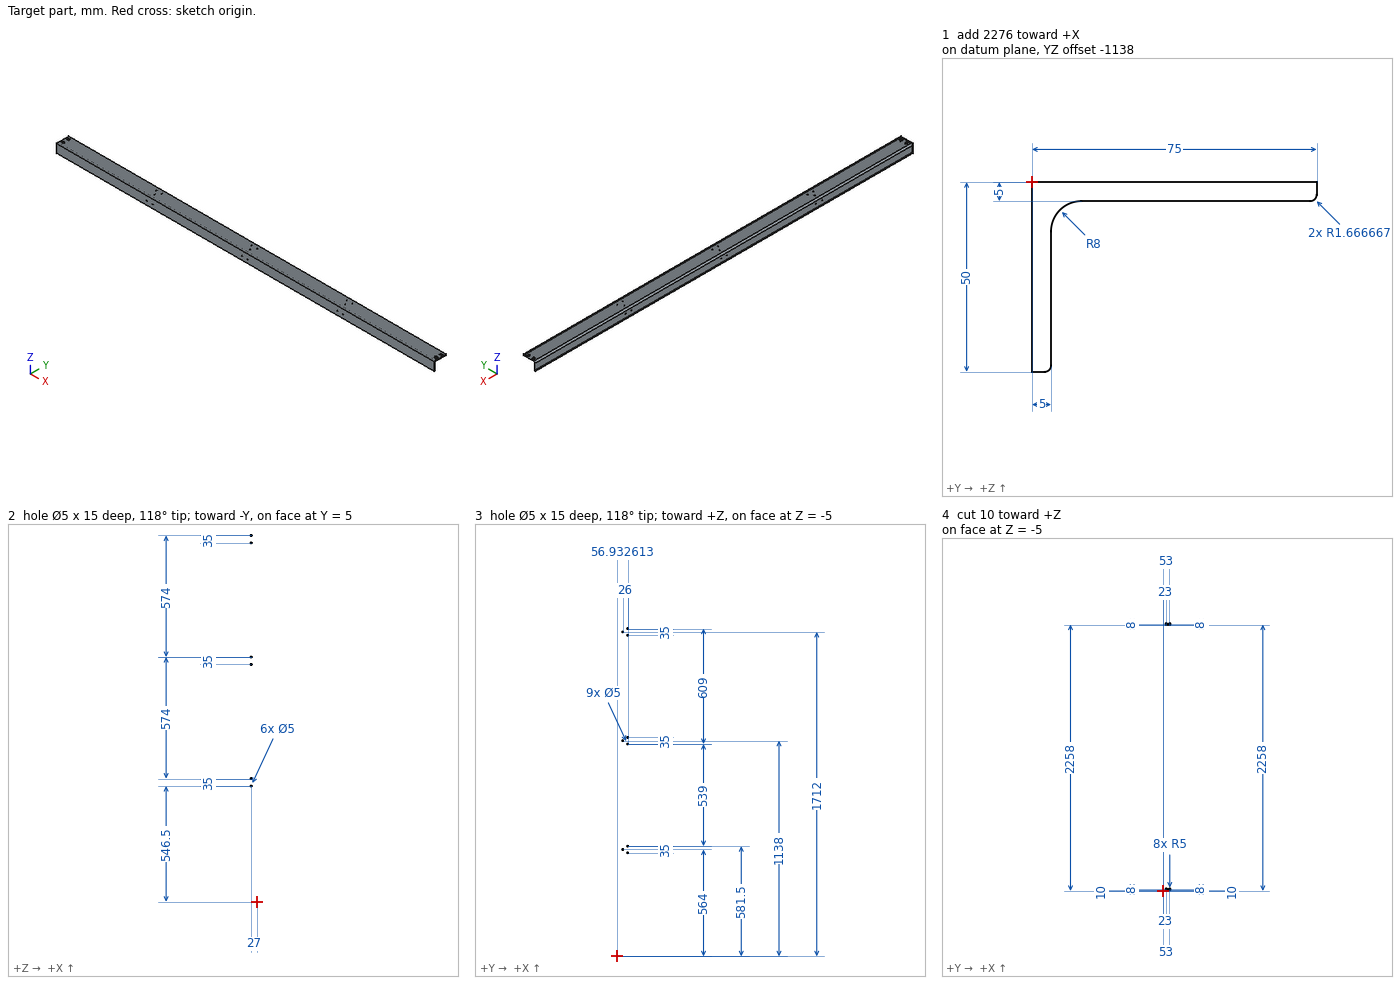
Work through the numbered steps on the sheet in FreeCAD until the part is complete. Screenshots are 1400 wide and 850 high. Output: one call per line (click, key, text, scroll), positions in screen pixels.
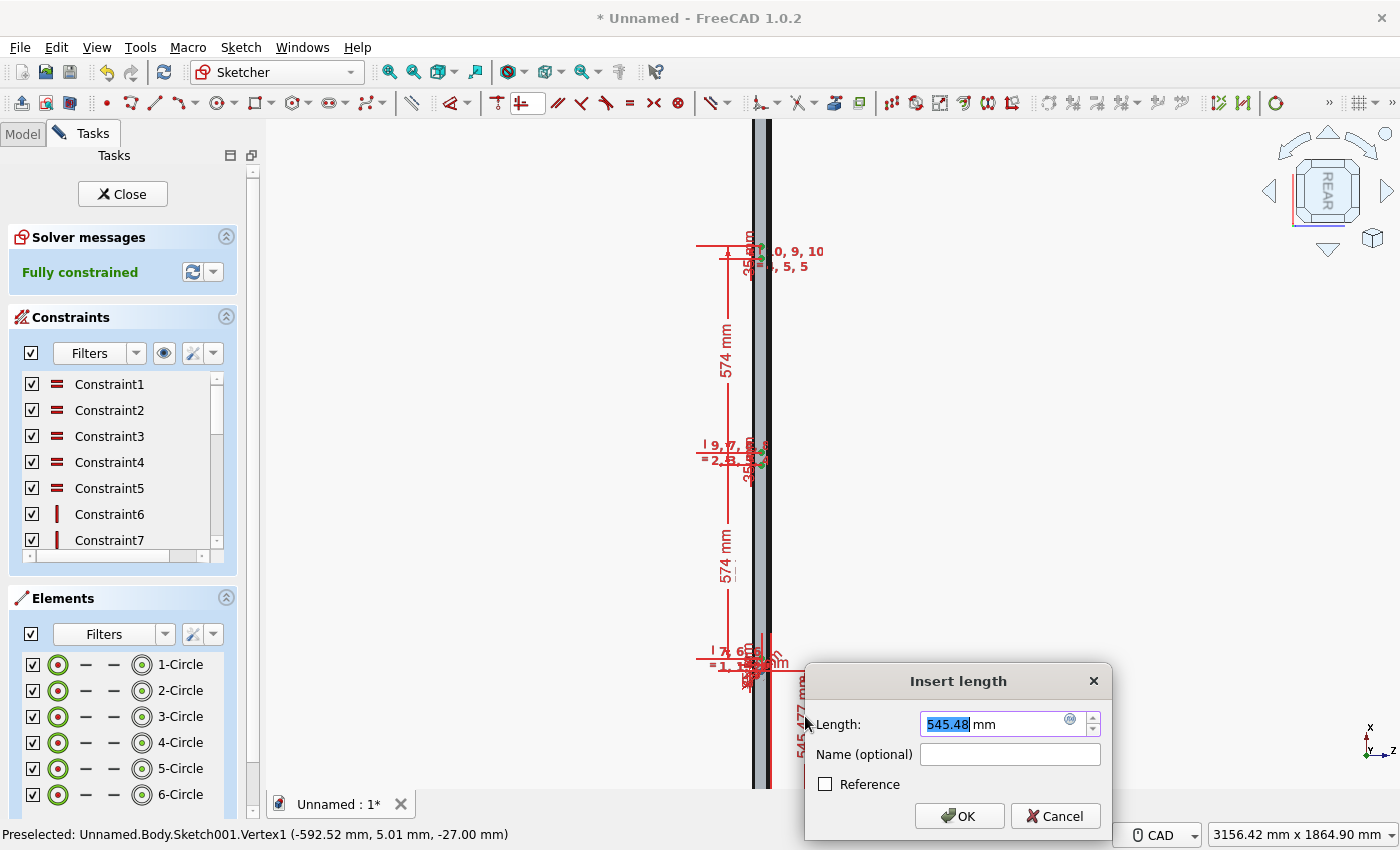
text(546.5)
key(Return)
key(Escape)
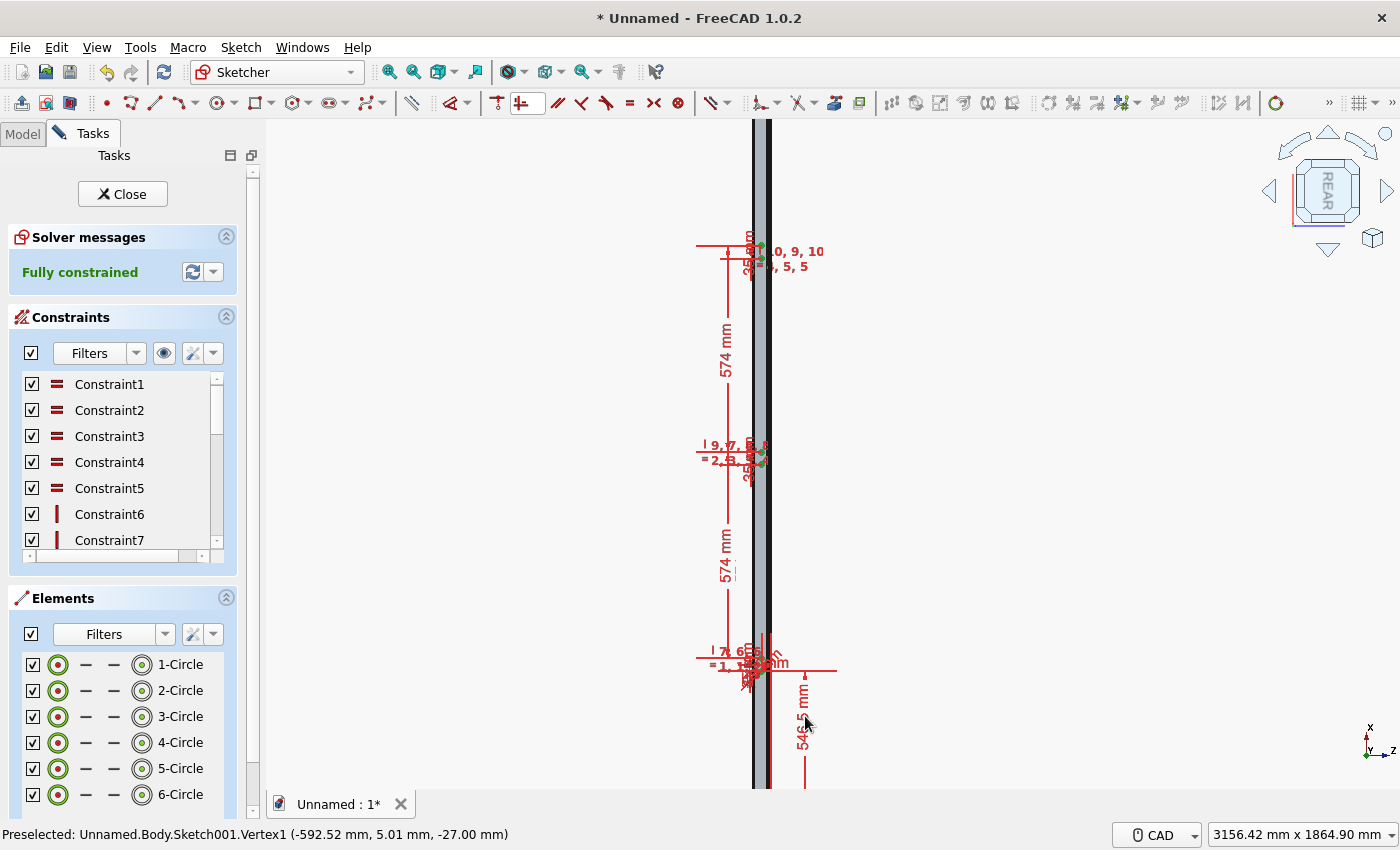
click(123, 194)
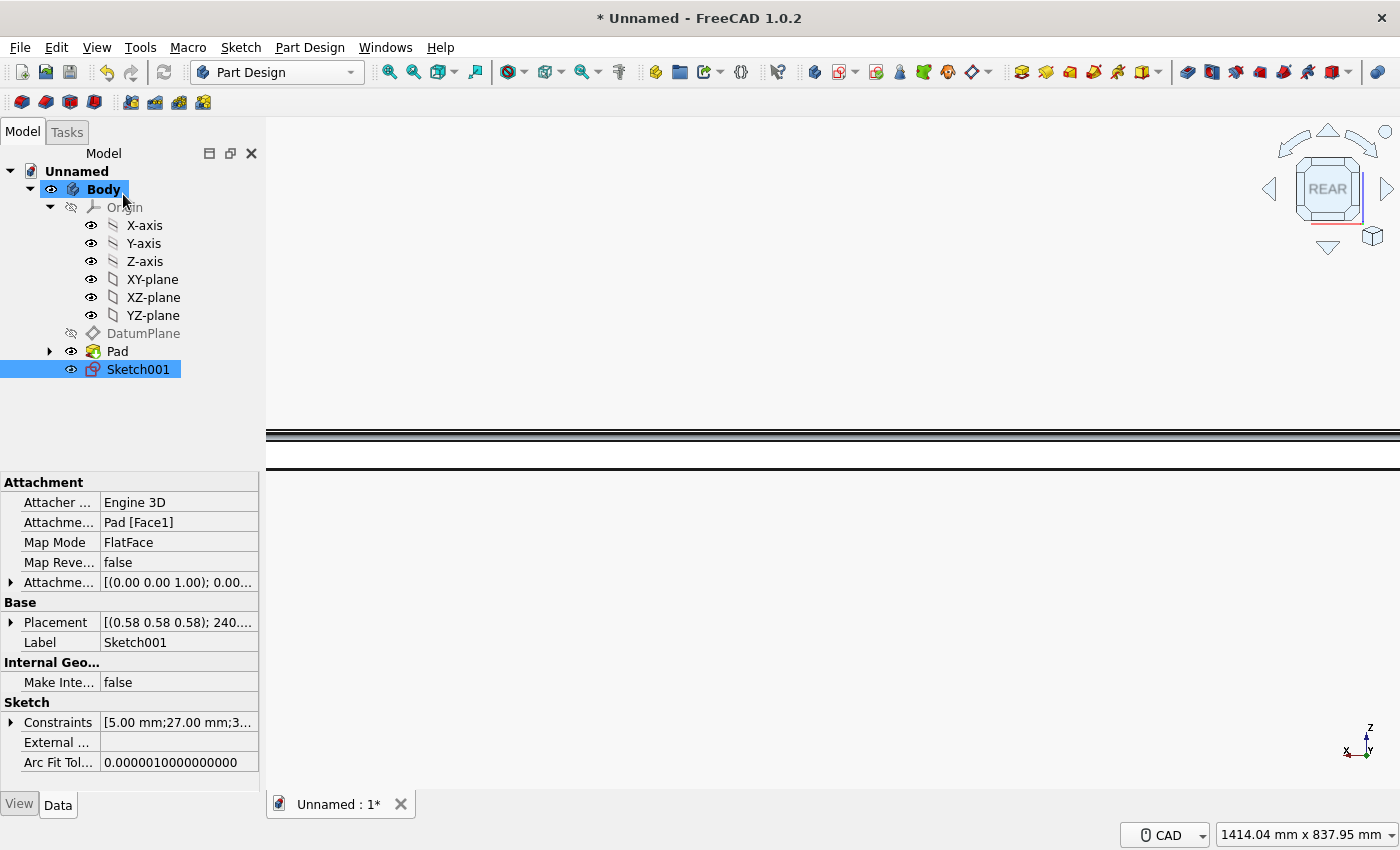
click(1212, 72)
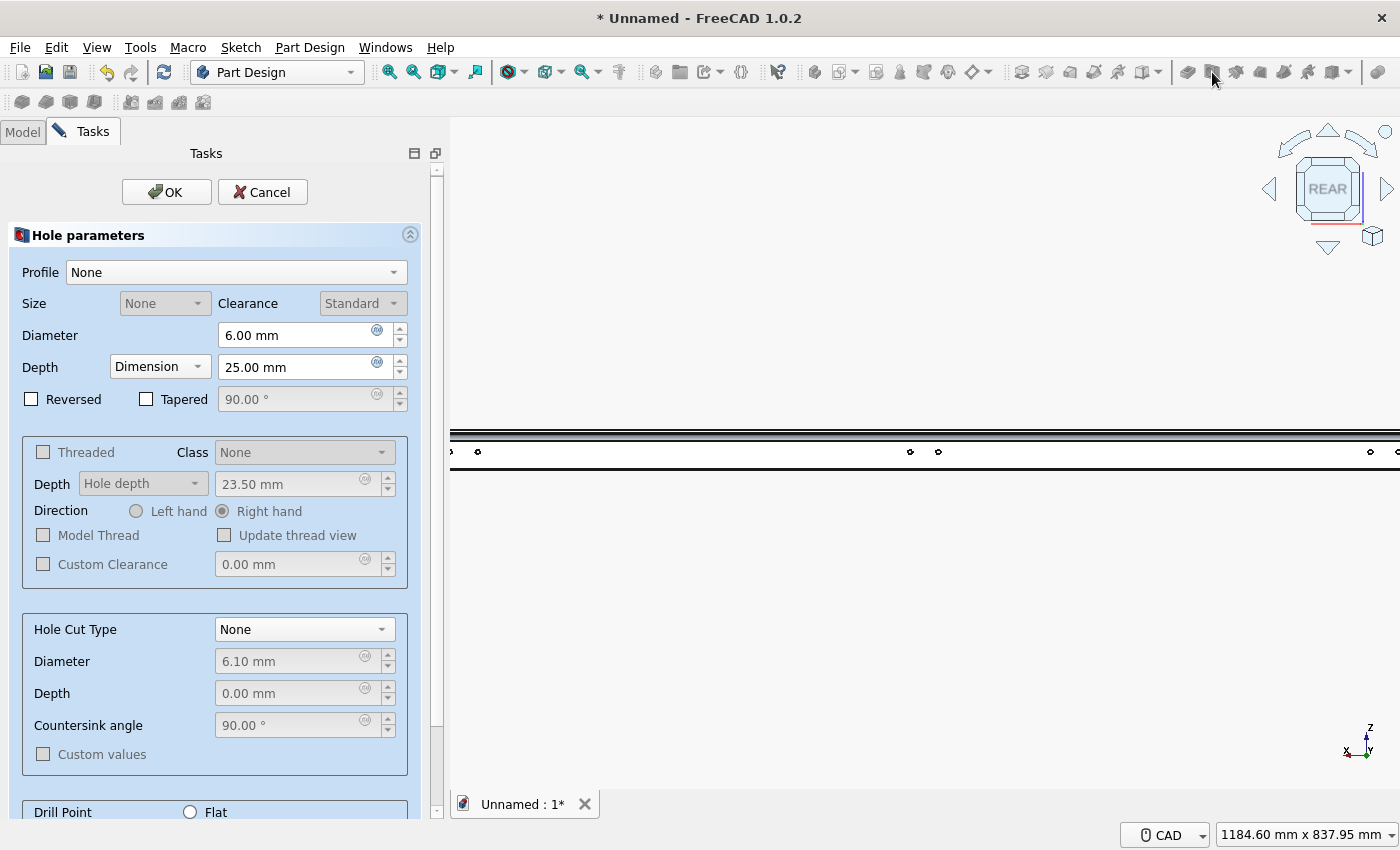
triple_click(305, 335)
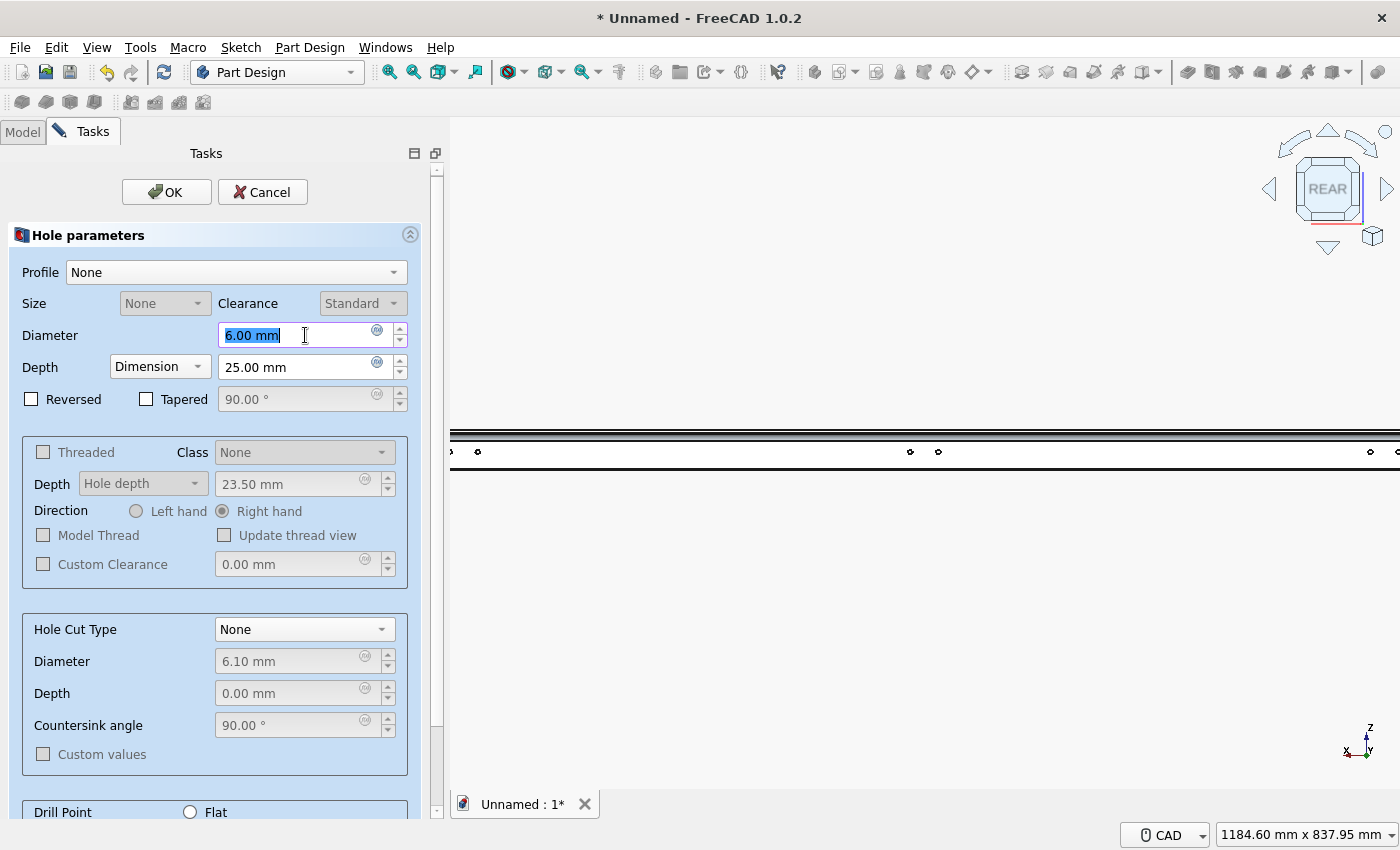
text(5)
key(Tab)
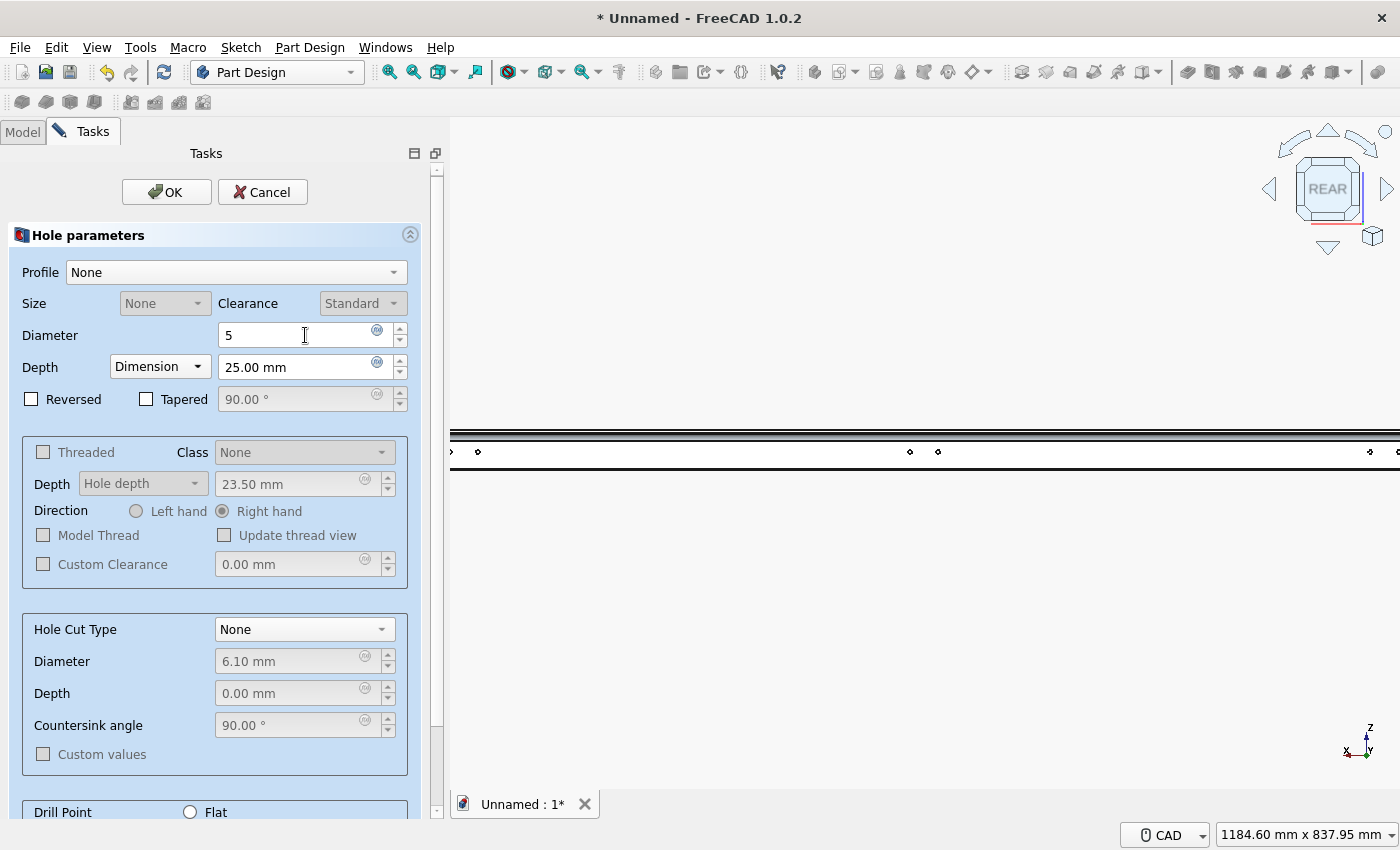
triple_click(305, 367)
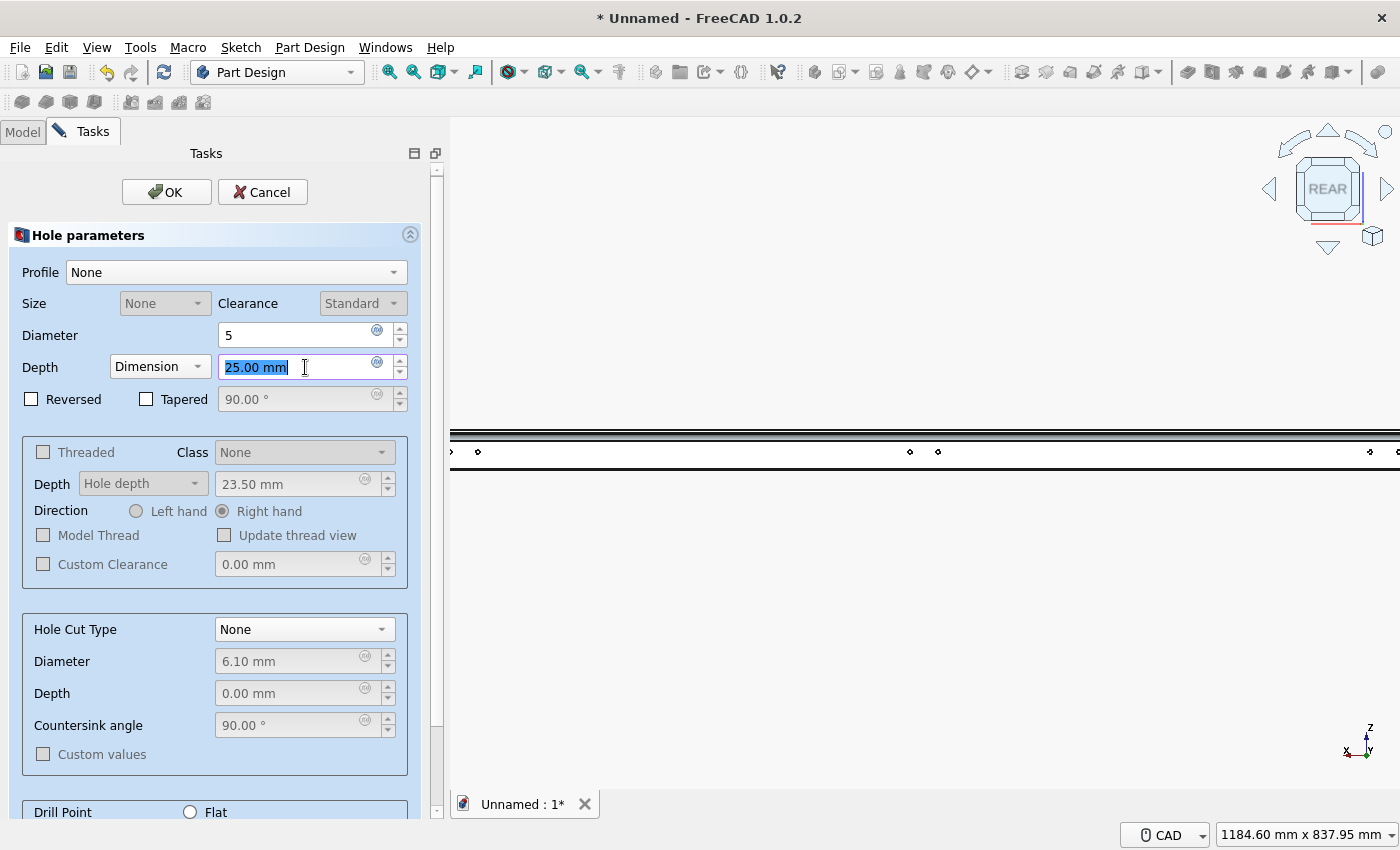
text(15)
key(Tab)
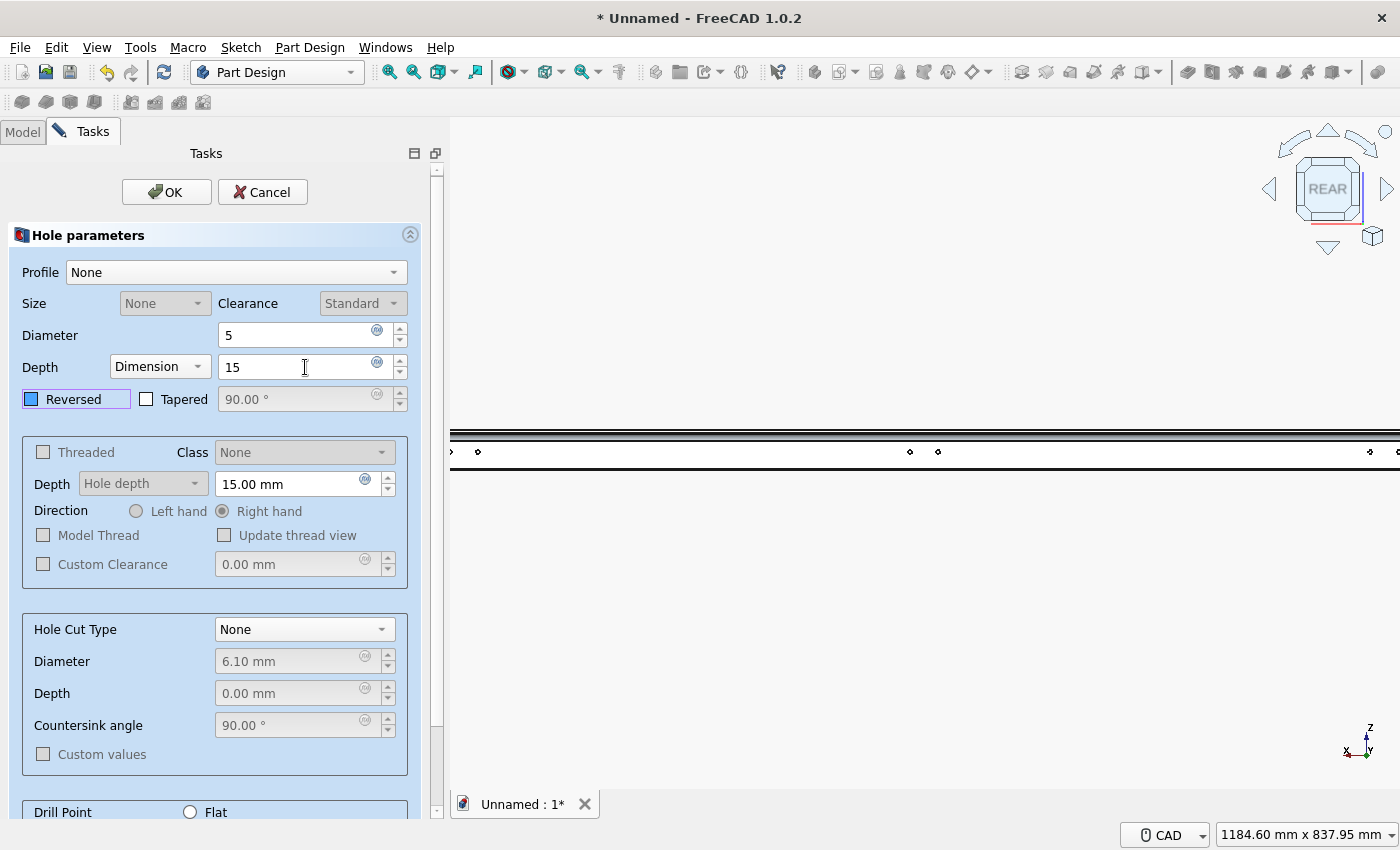
click(167, 192)